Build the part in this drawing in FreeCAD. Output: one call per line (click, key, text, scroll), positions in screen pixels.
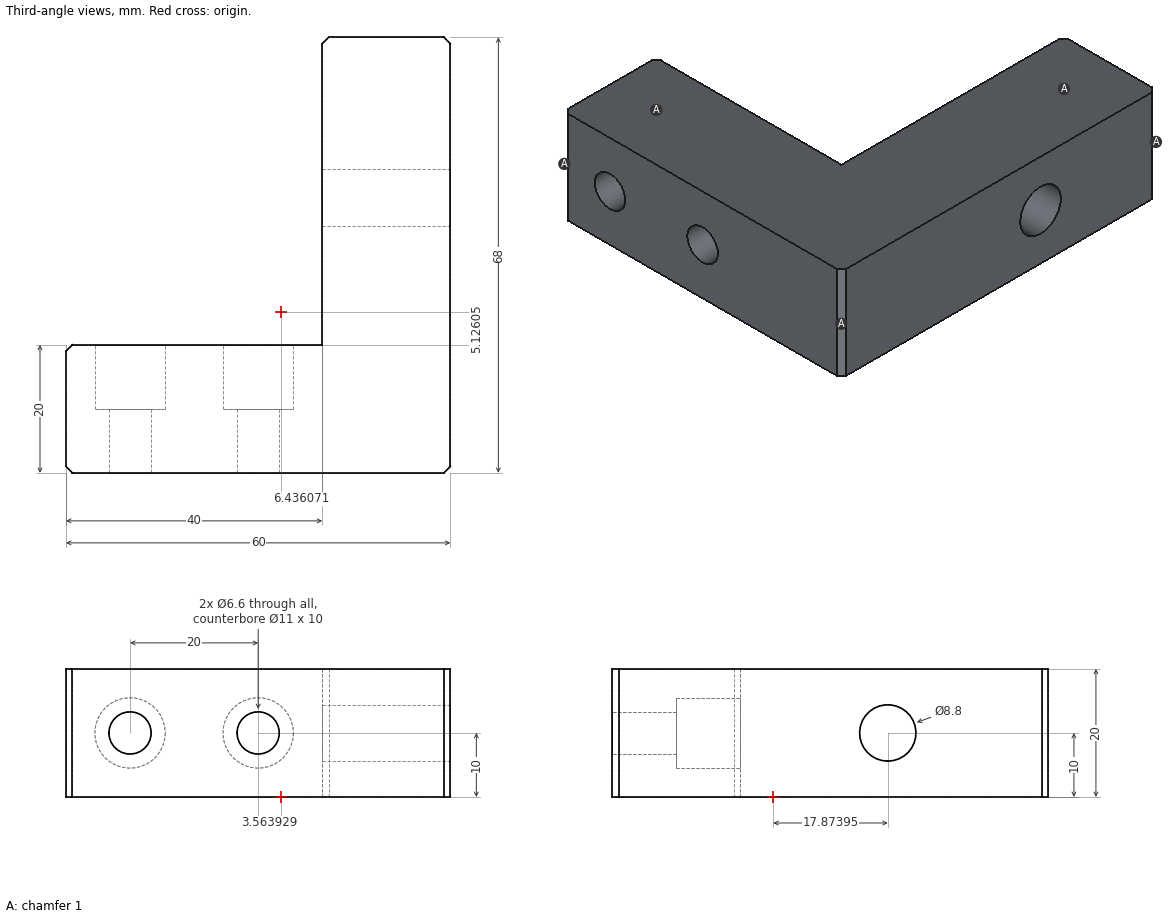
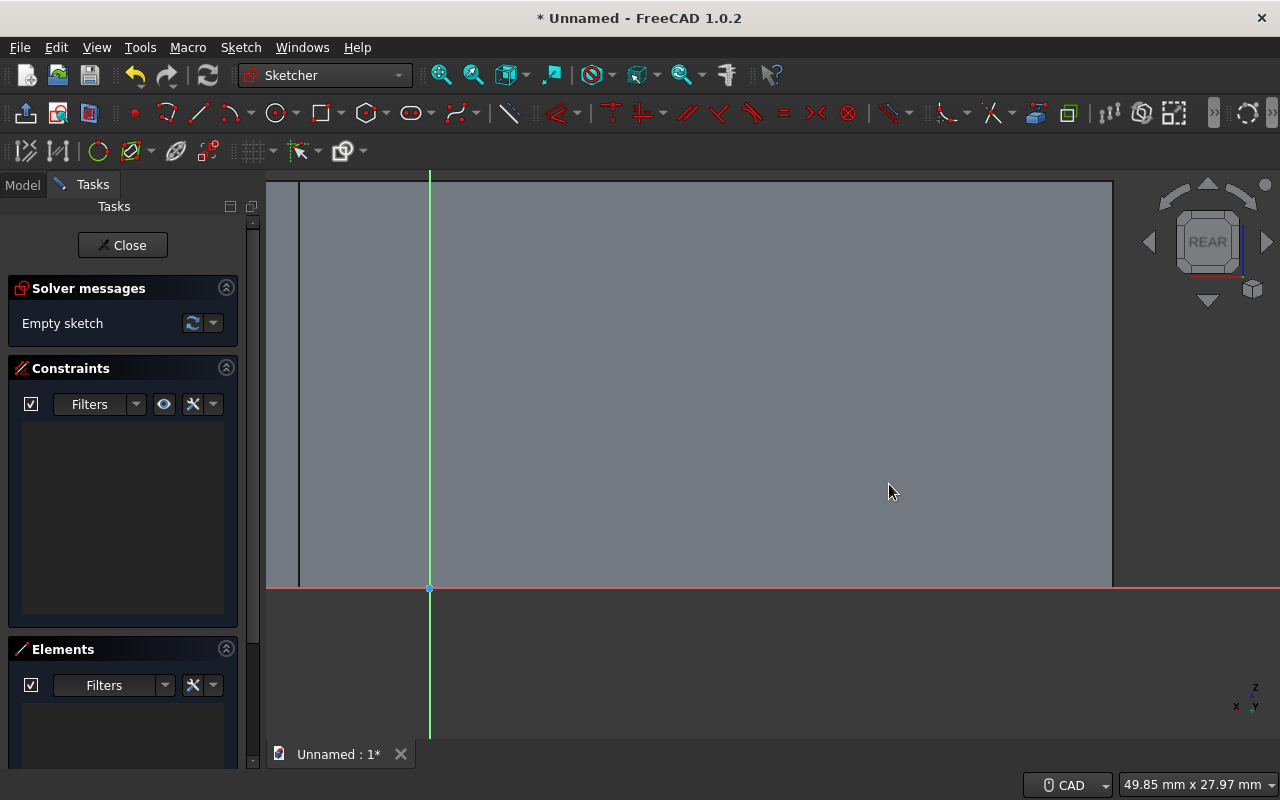
click(276, 114)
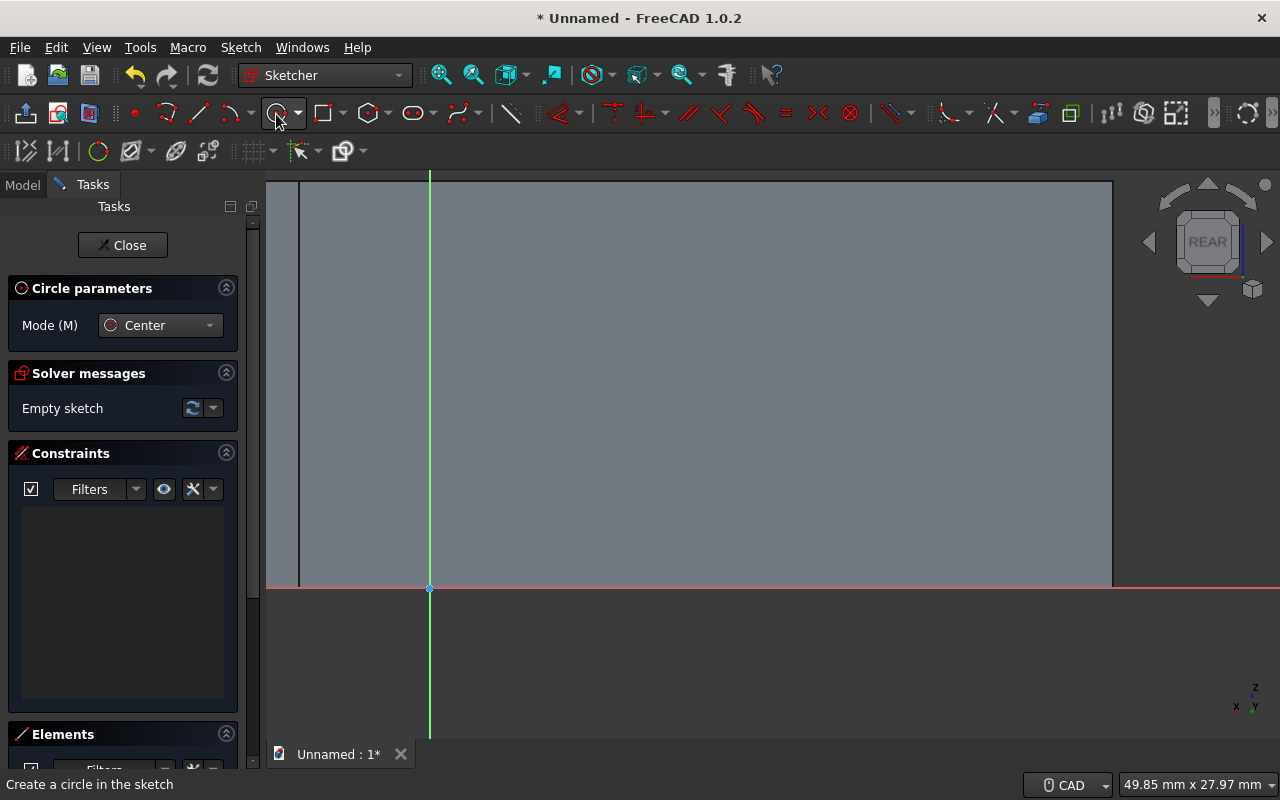
click(502, 385)
move(550, 337)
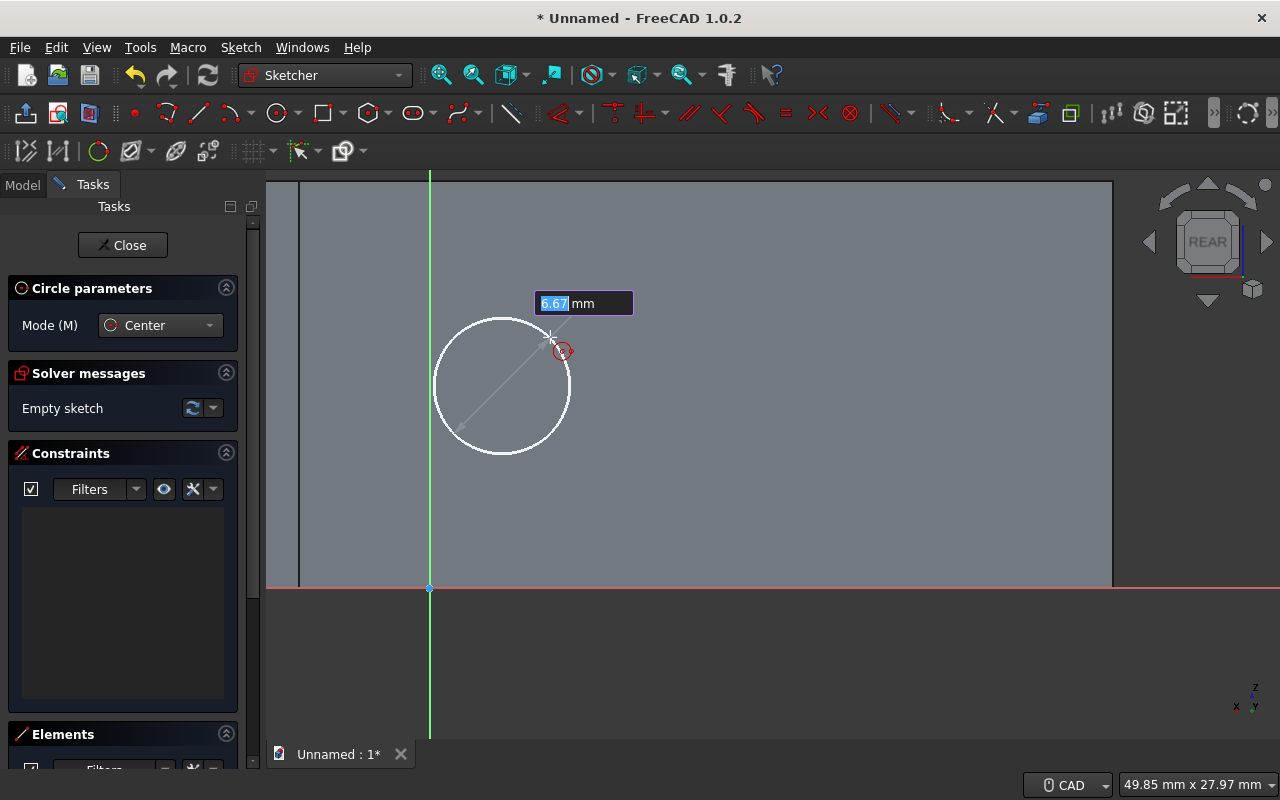
text(6.6)
key(Return)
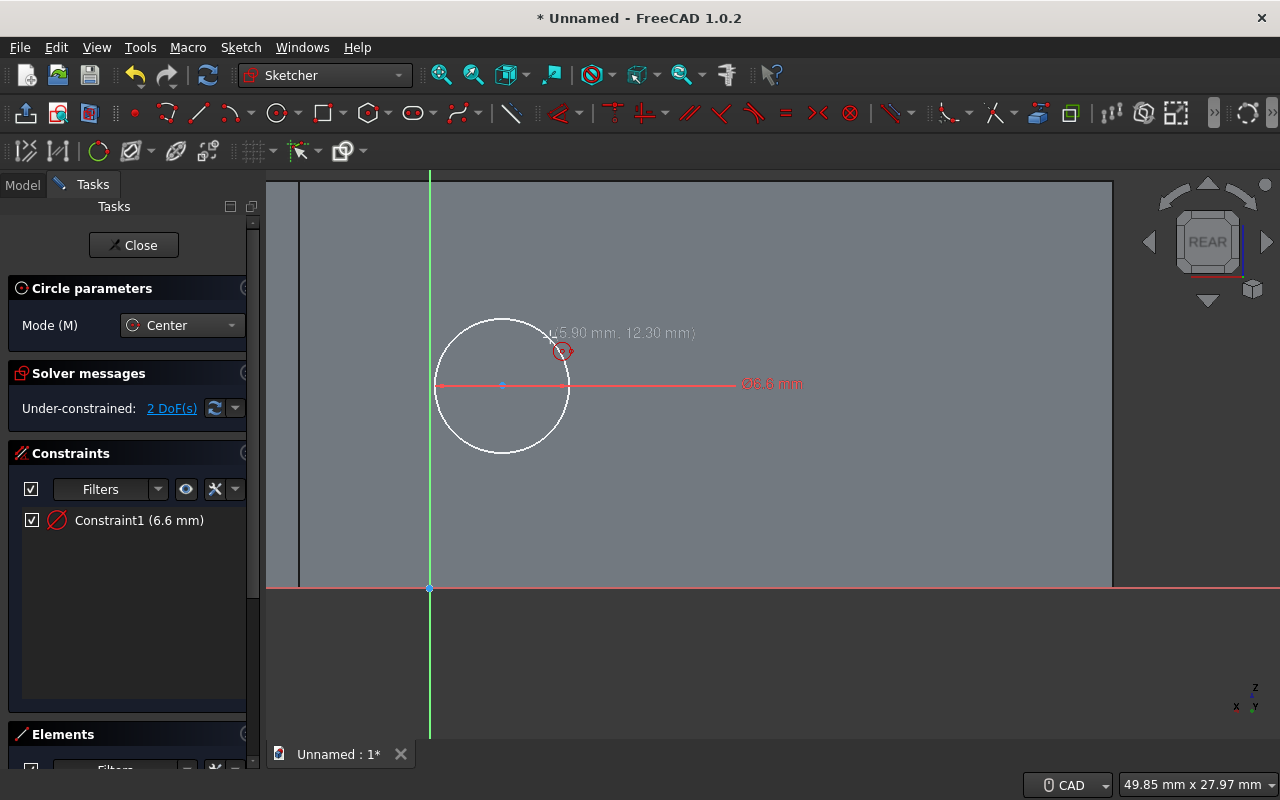
click(909, 385)
move(957, 337)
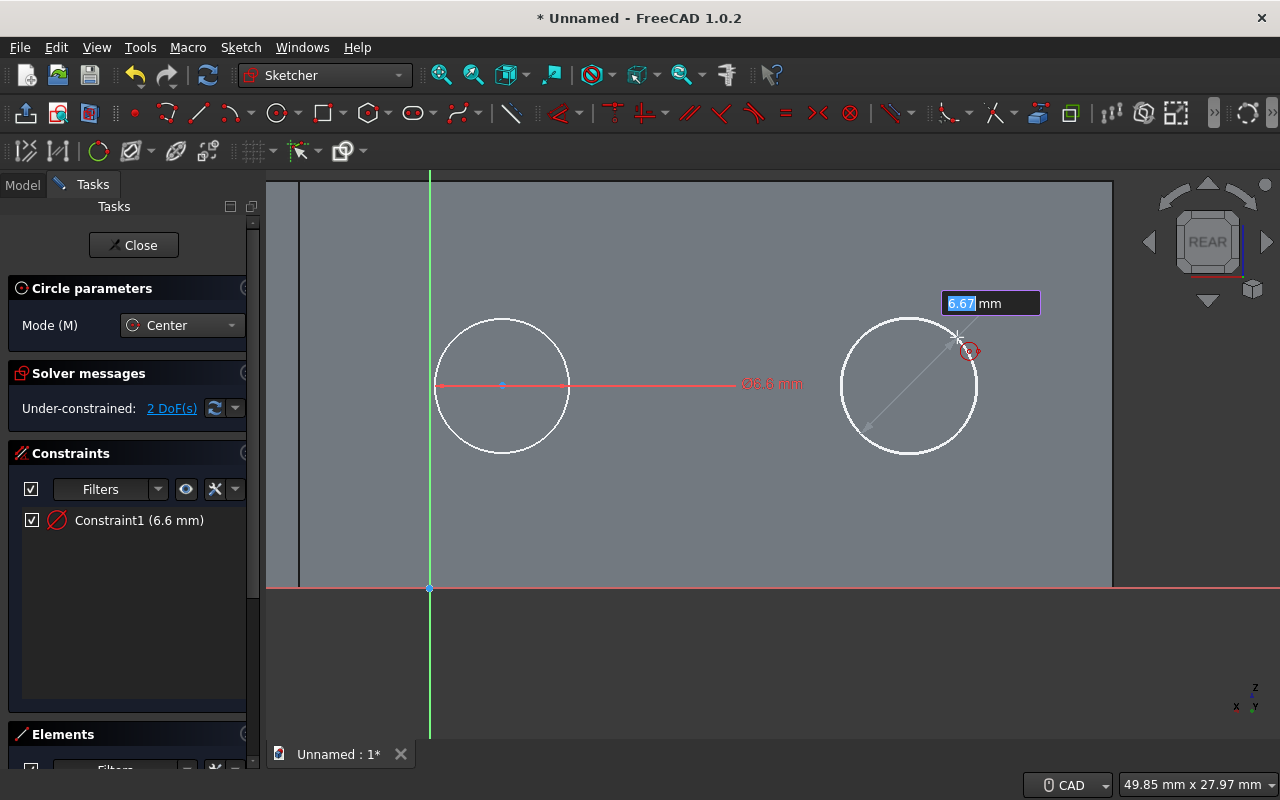
text(6.6)
key(Return)
key(Escape)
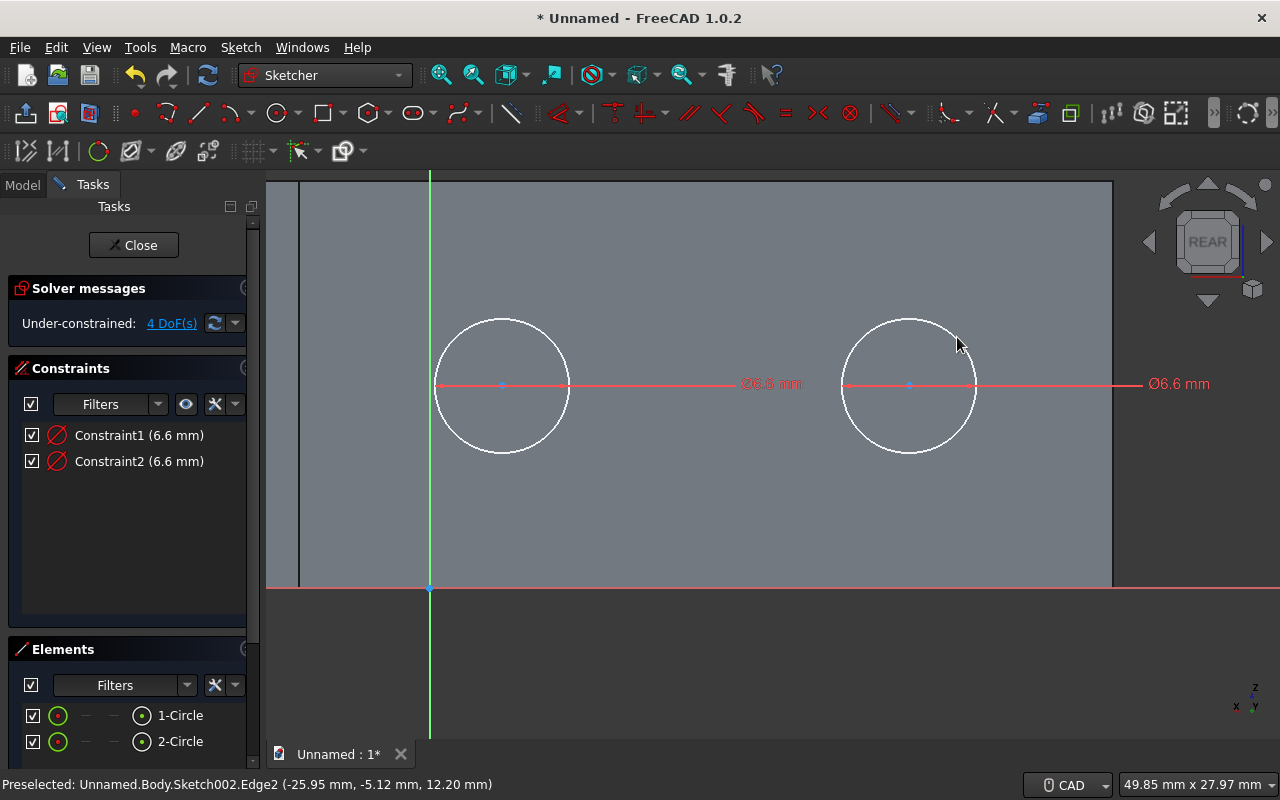
click(502, 386)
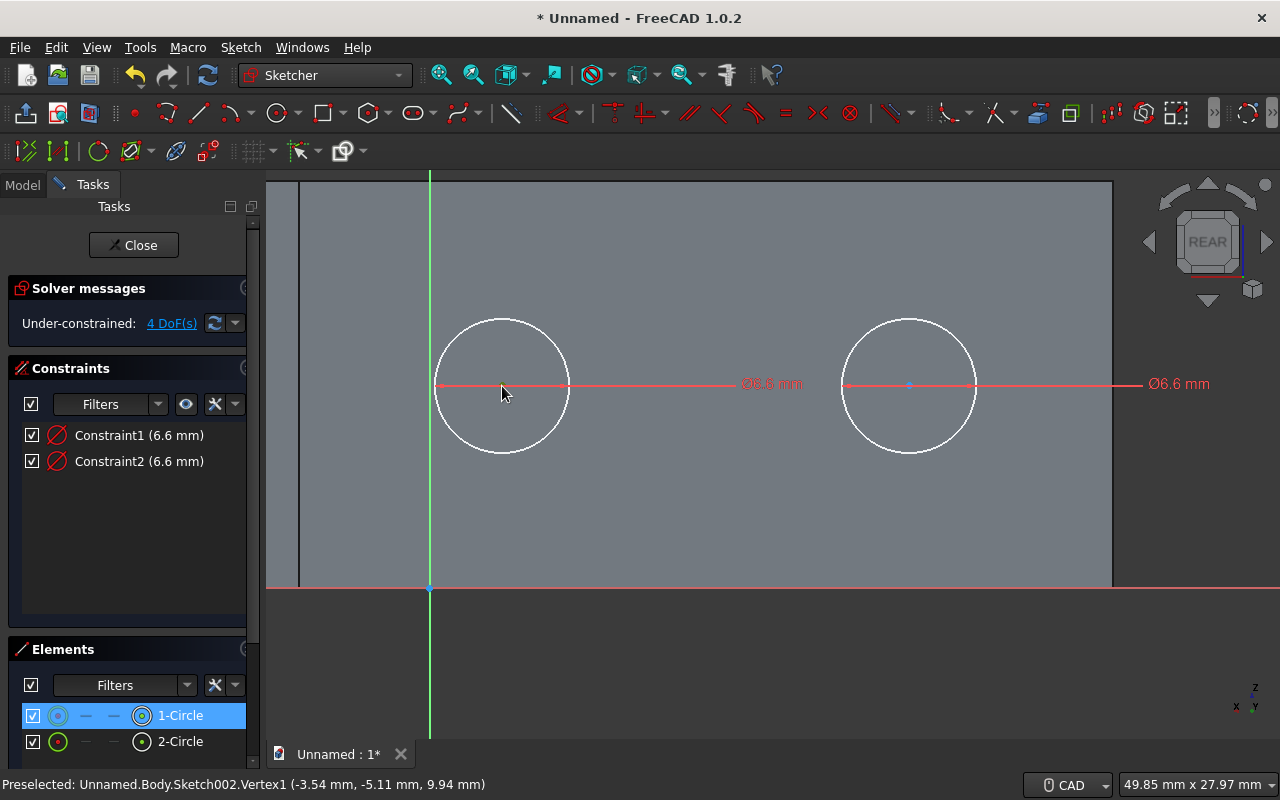
click(909, 386)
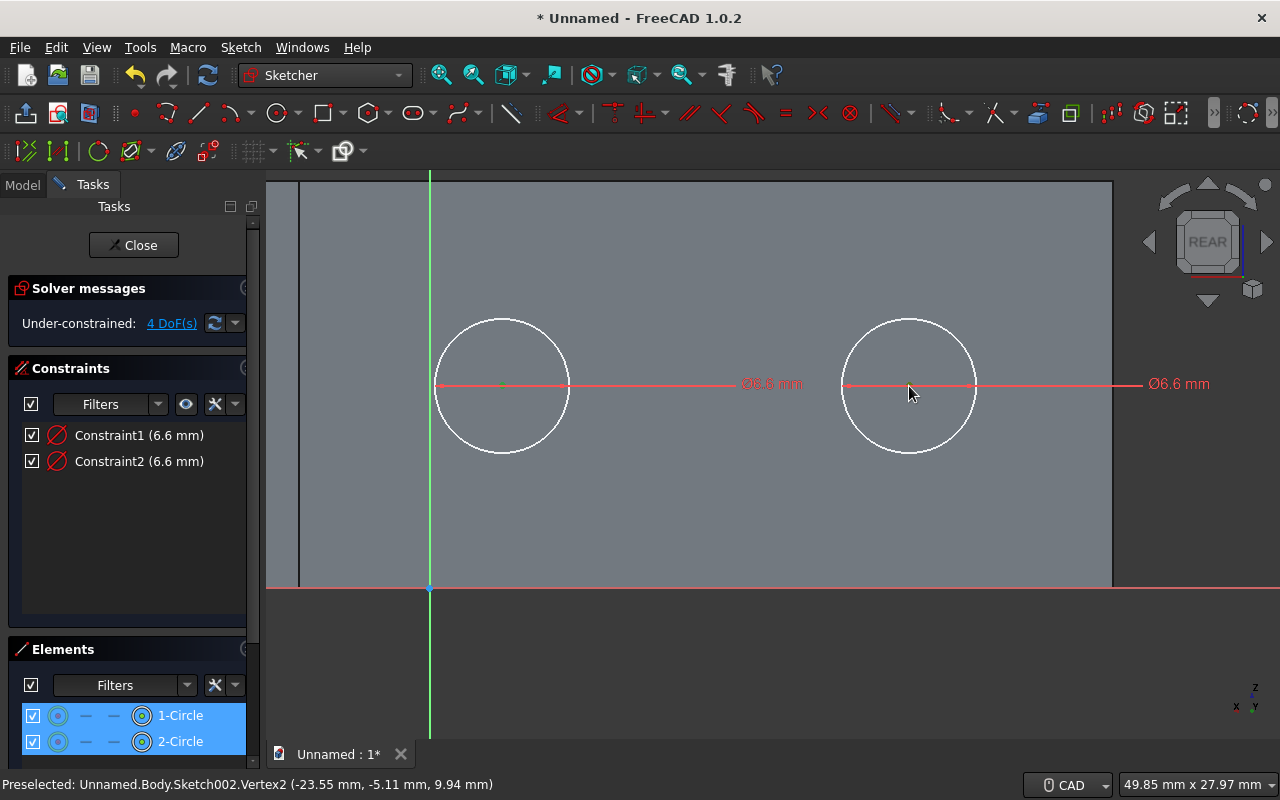
click(668, 114)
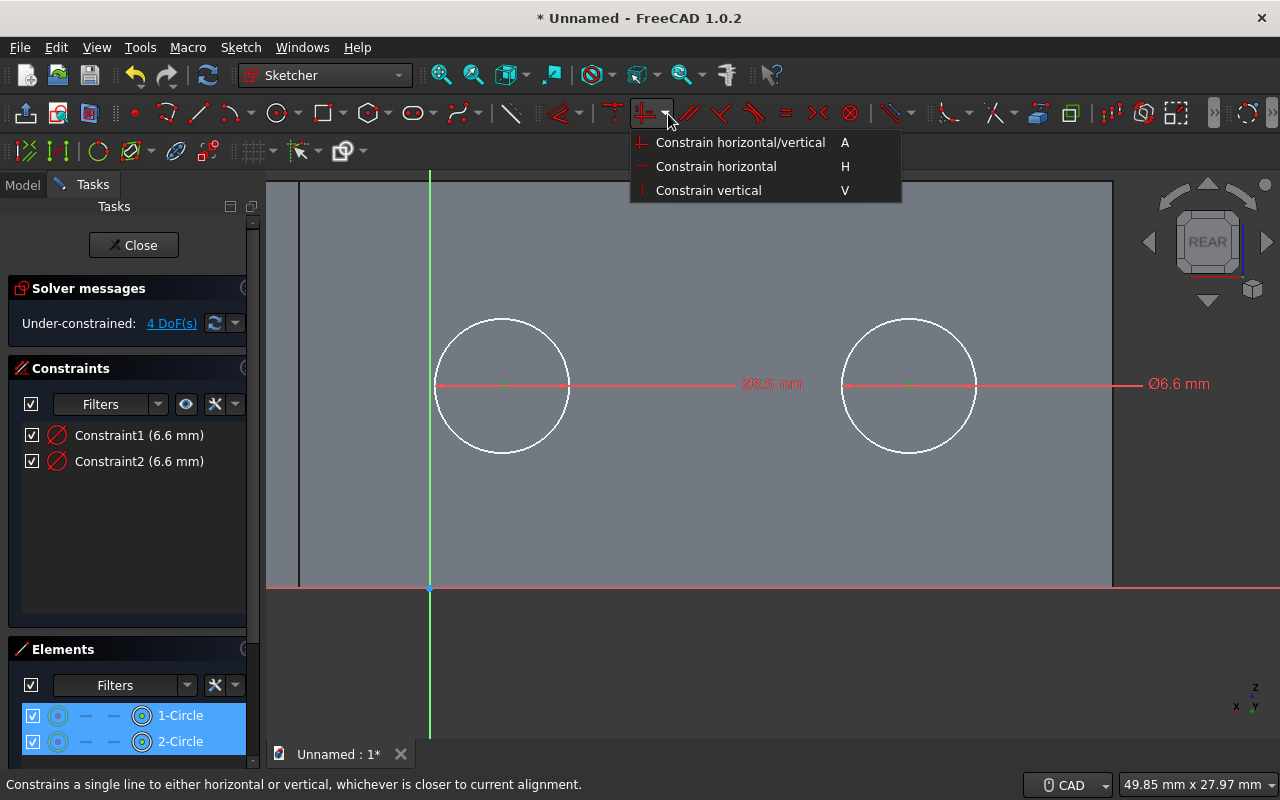
click(766, 166)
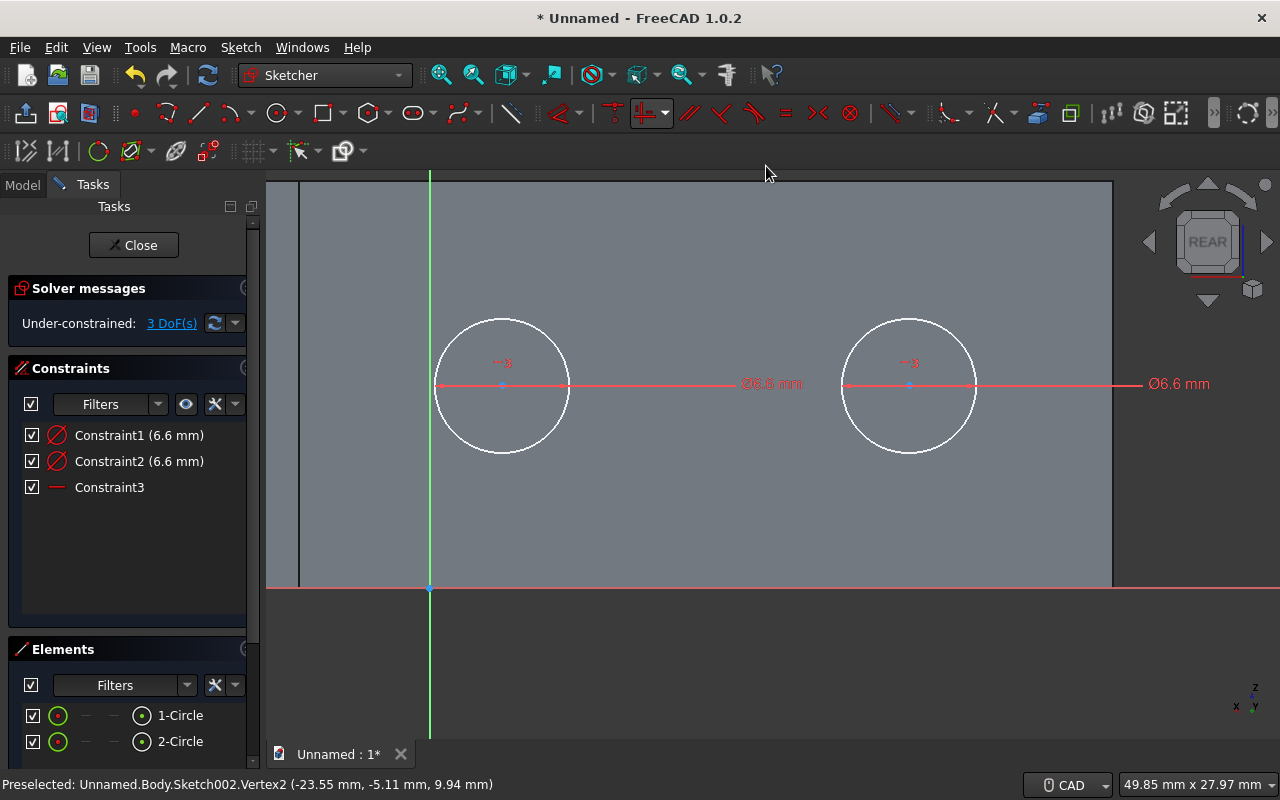
key(d)